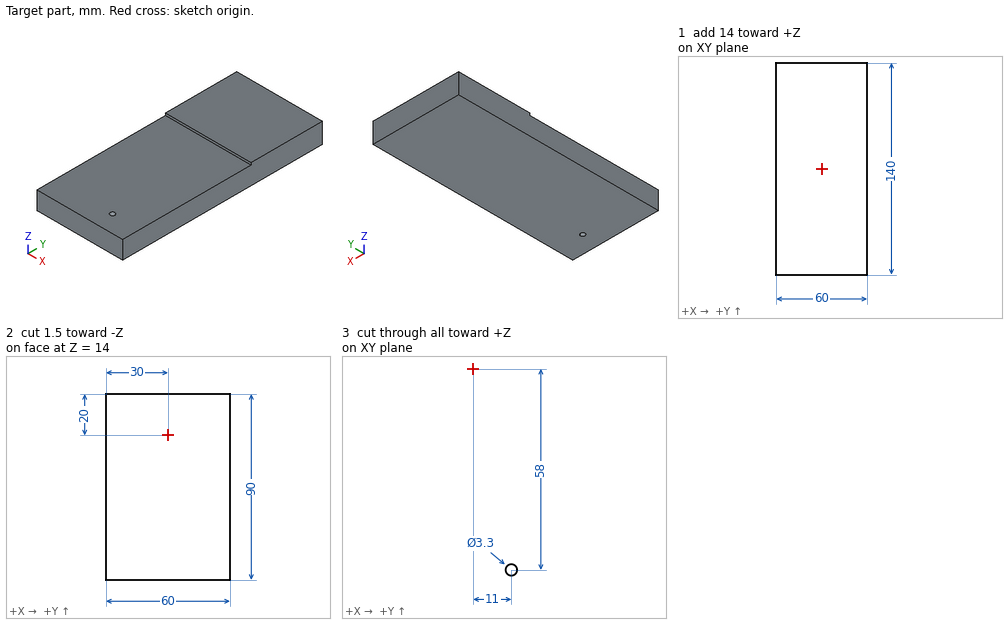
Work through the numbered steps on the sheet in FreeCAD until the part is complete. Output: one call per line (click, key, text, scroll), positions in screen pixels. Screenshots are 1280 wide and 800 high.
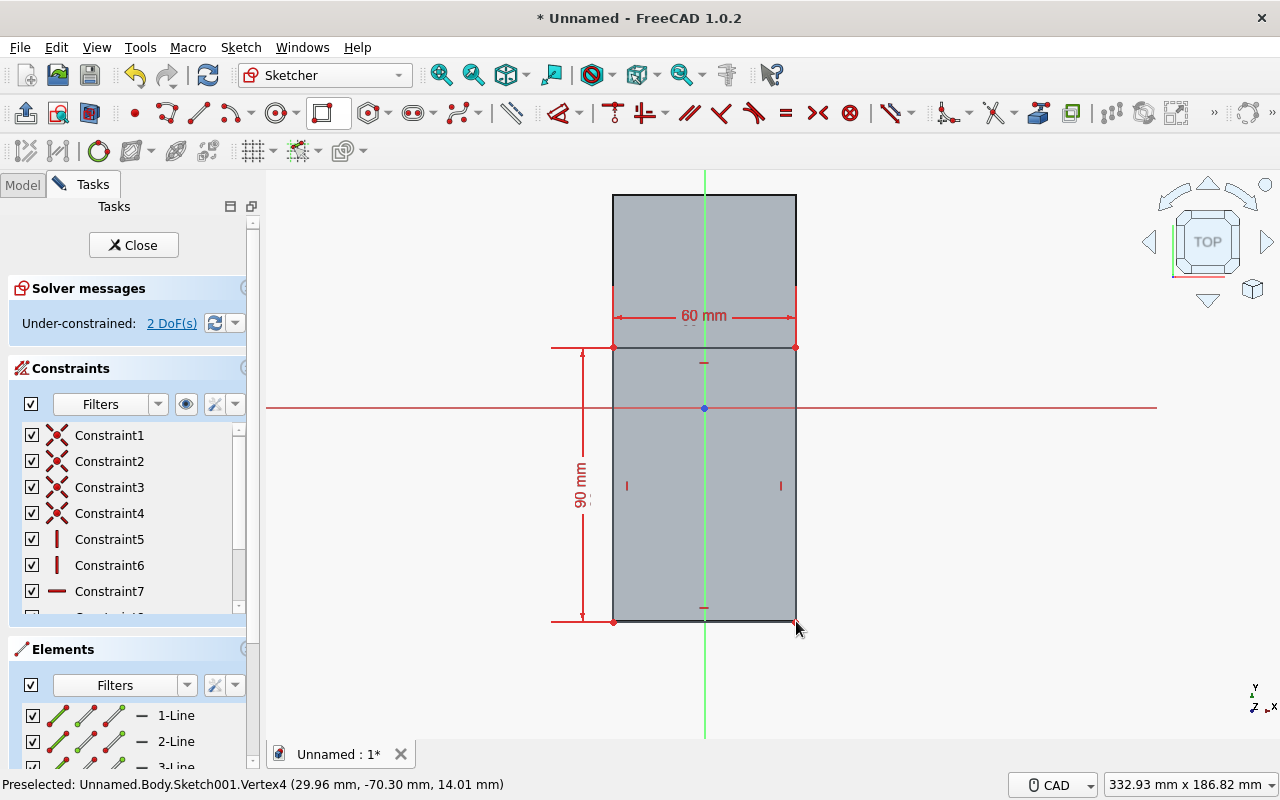
click(558, 114)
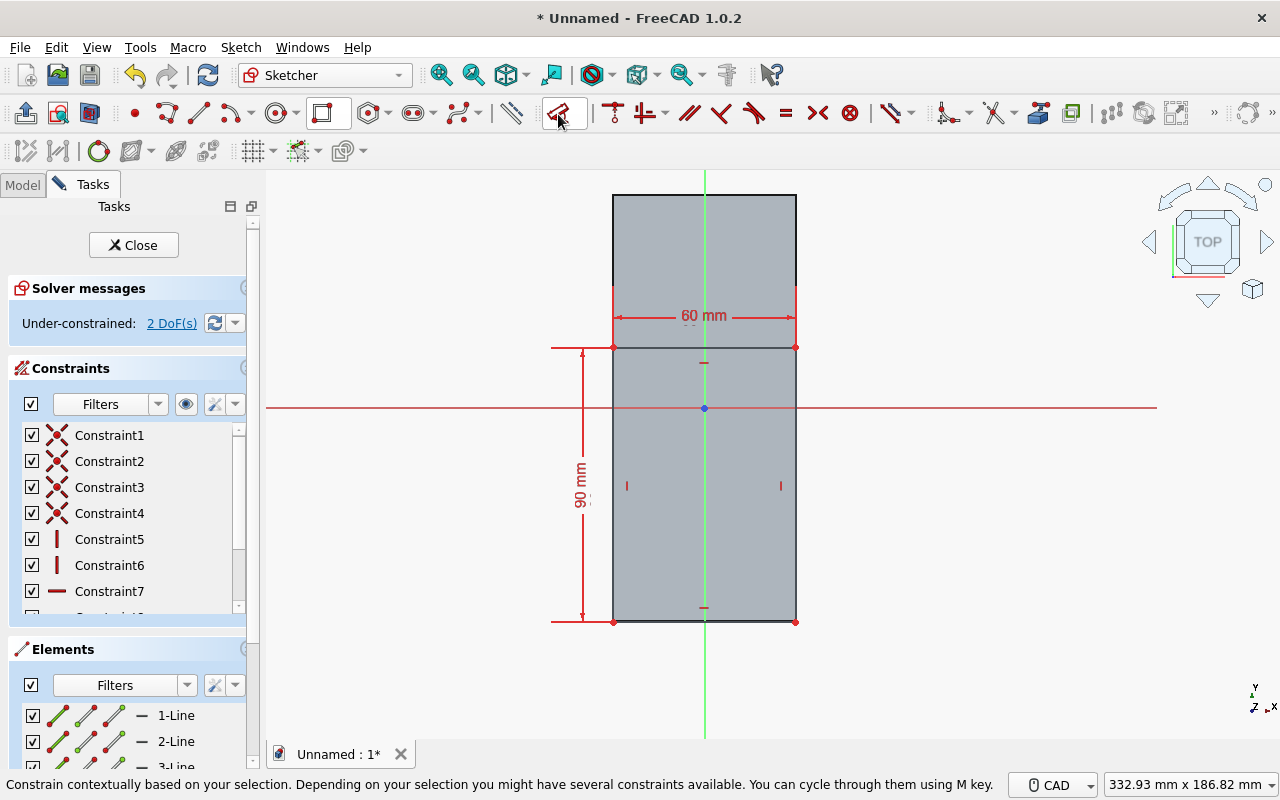
click(613, 348)
click(659, 314)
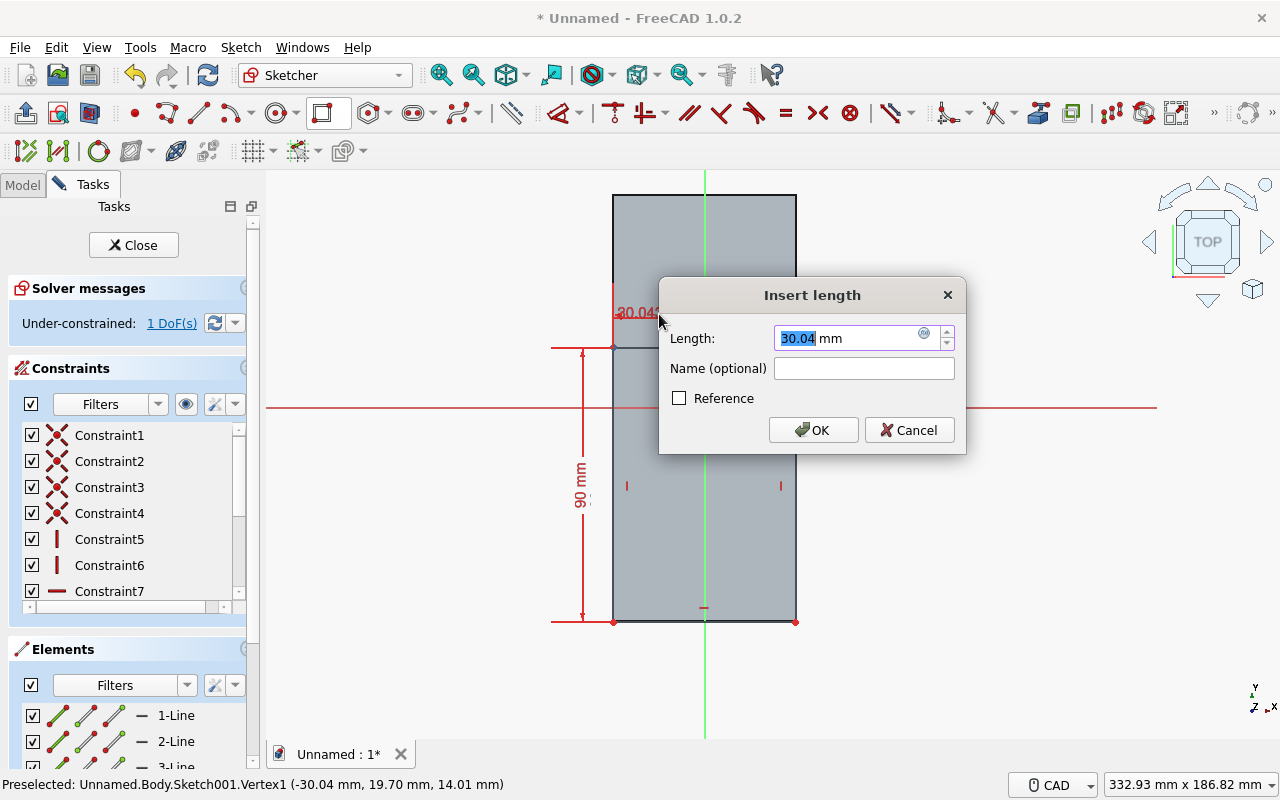
text(30)
key(Return)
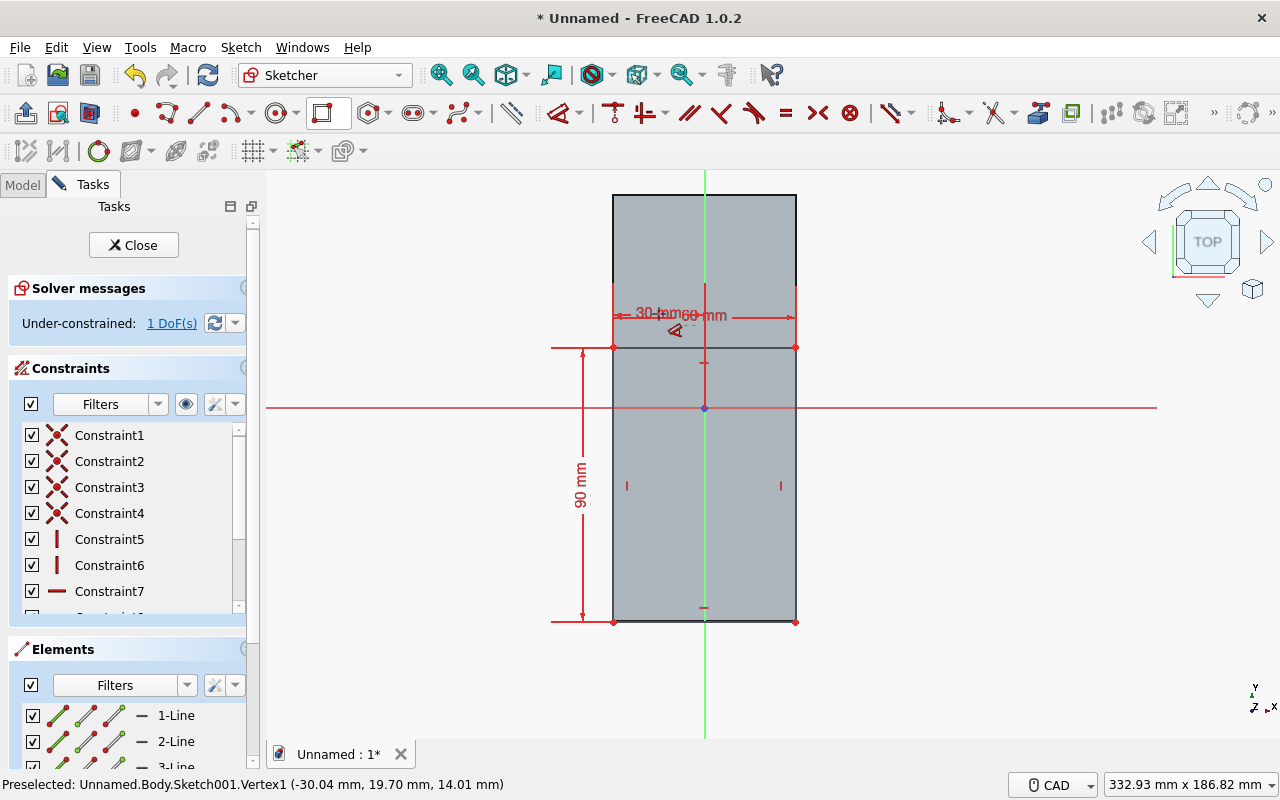
click(613, 348)
click(579, 378)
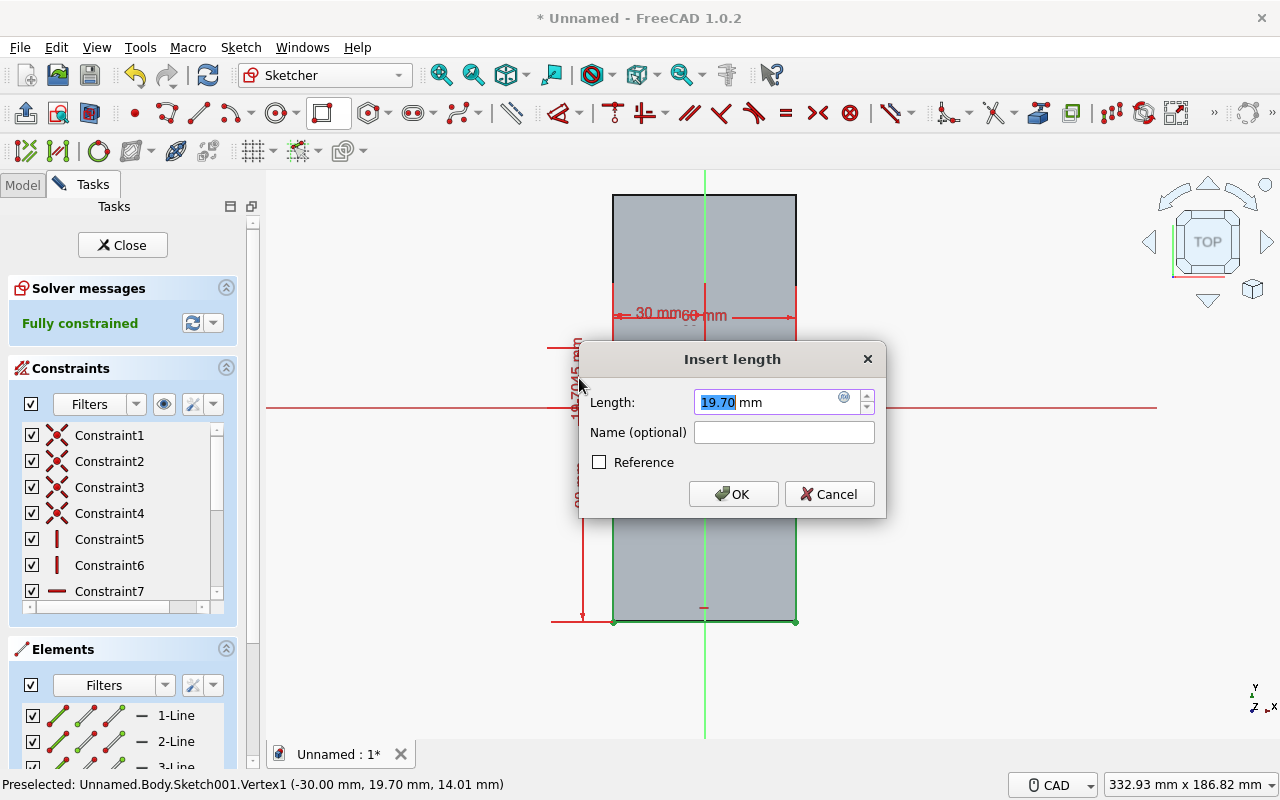
text(20)
key(Return)
key(Escape)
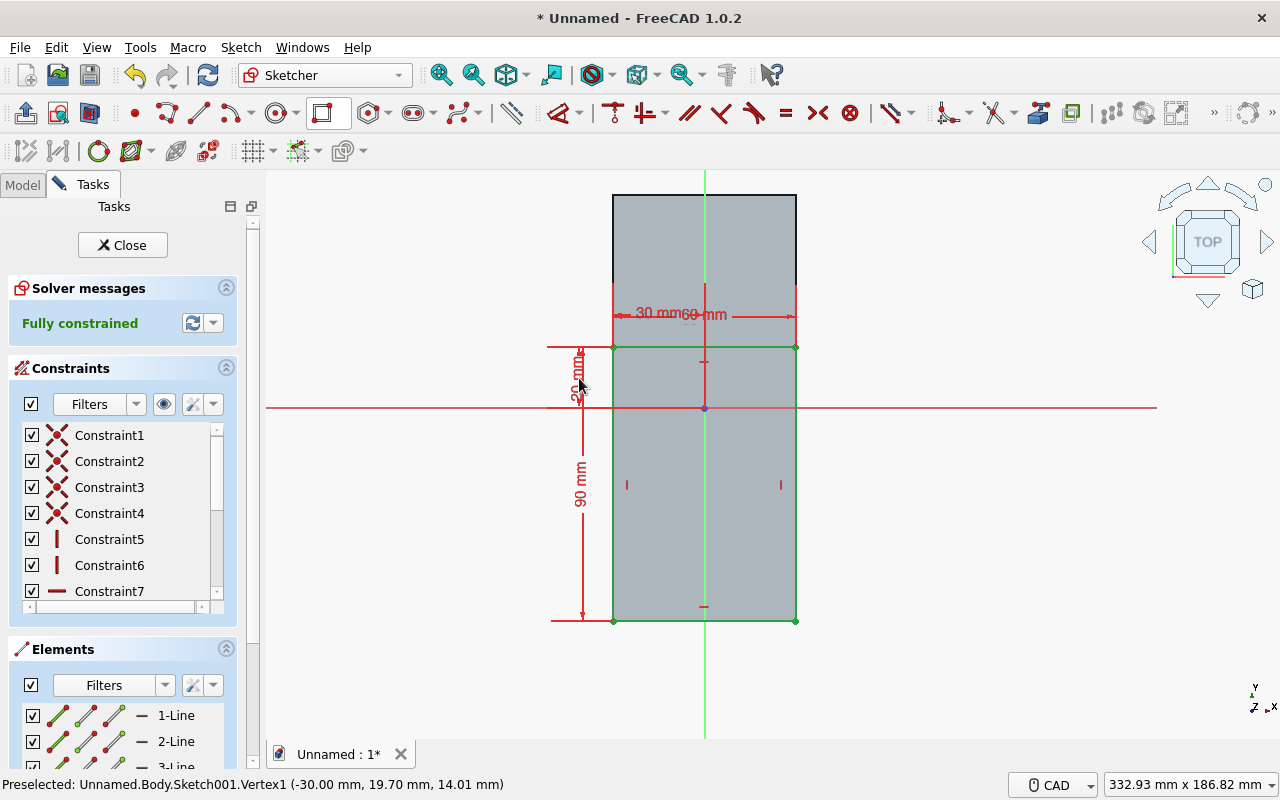
click(123, 245)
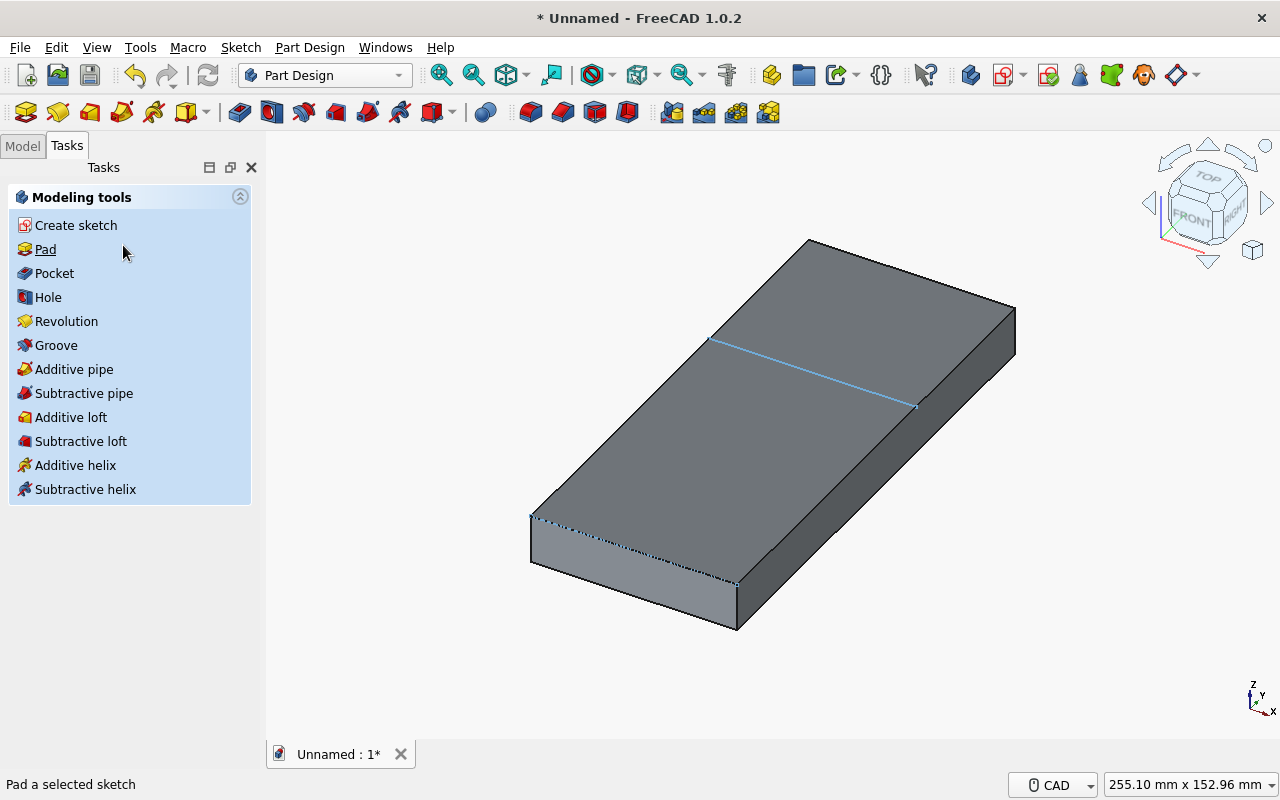
click(240, 112)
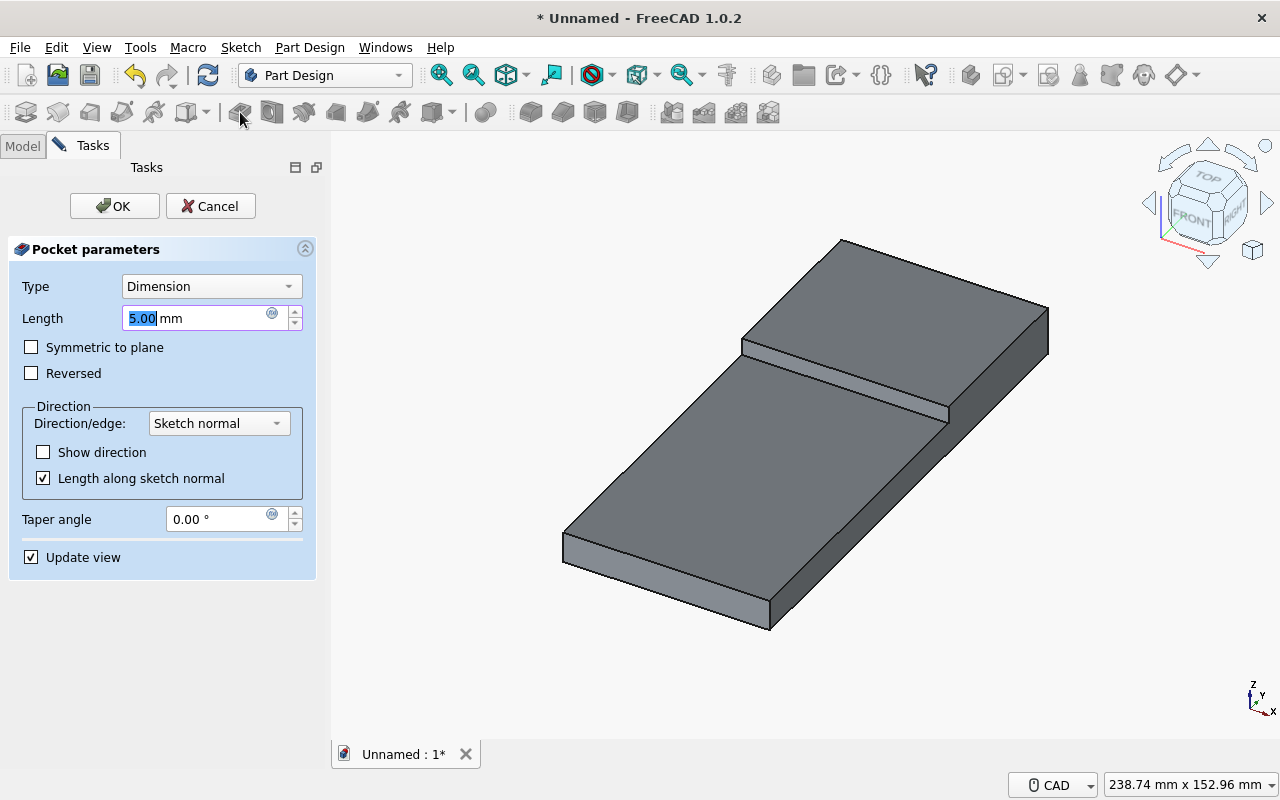
text(1.5)
key(Tab)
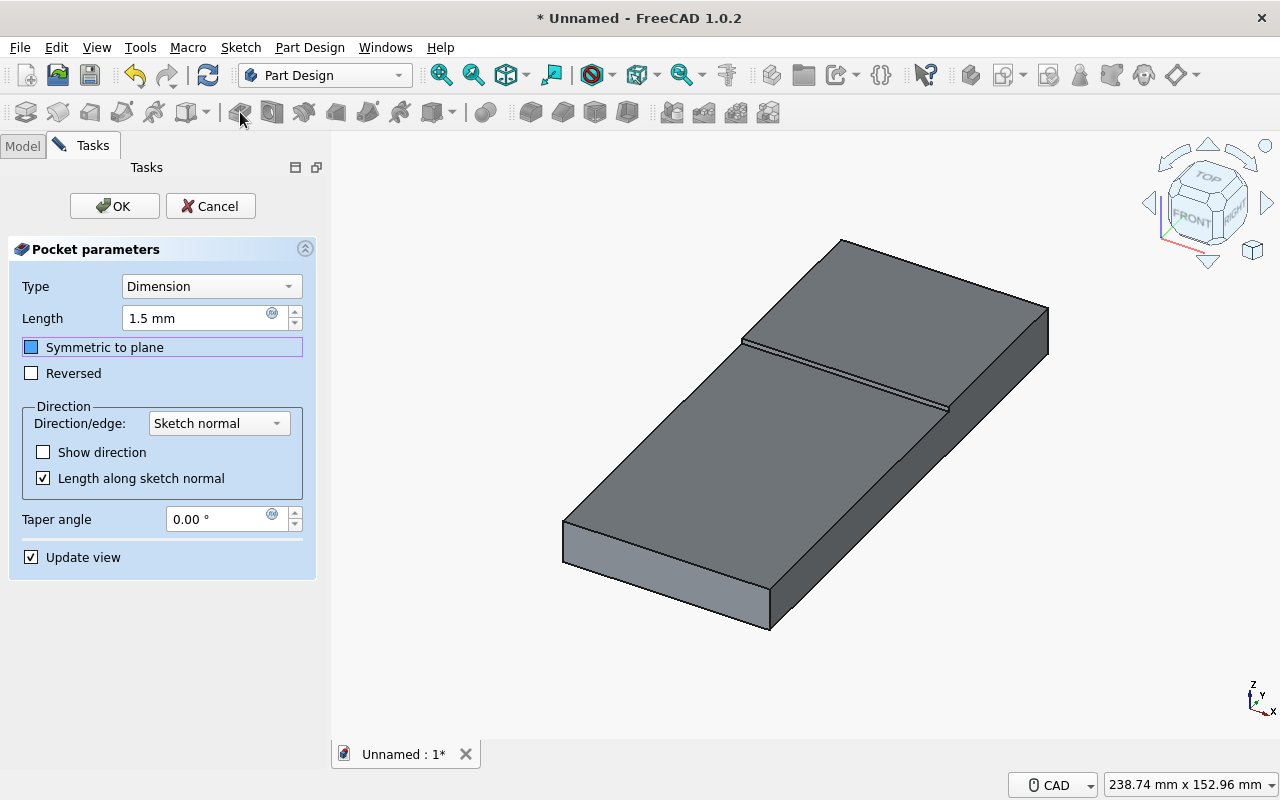
click(115, 206)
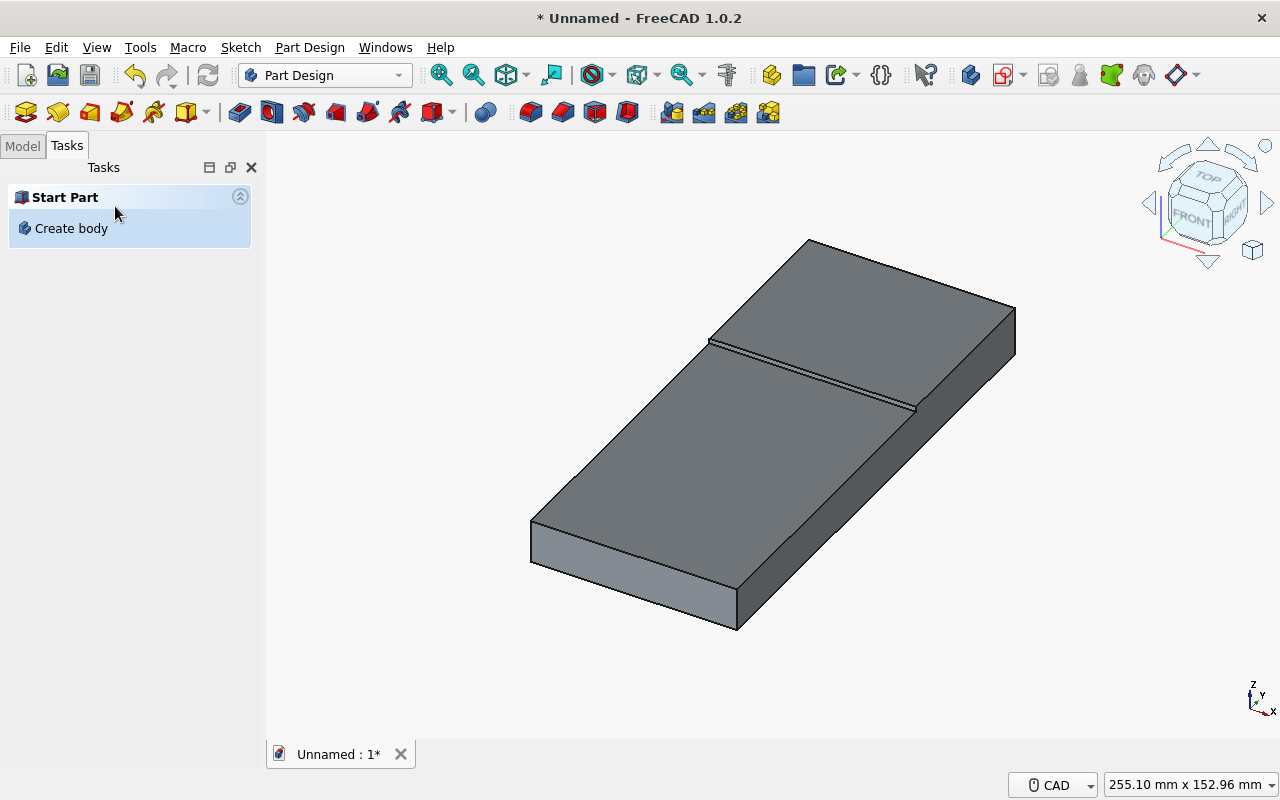
click(1004, 76)